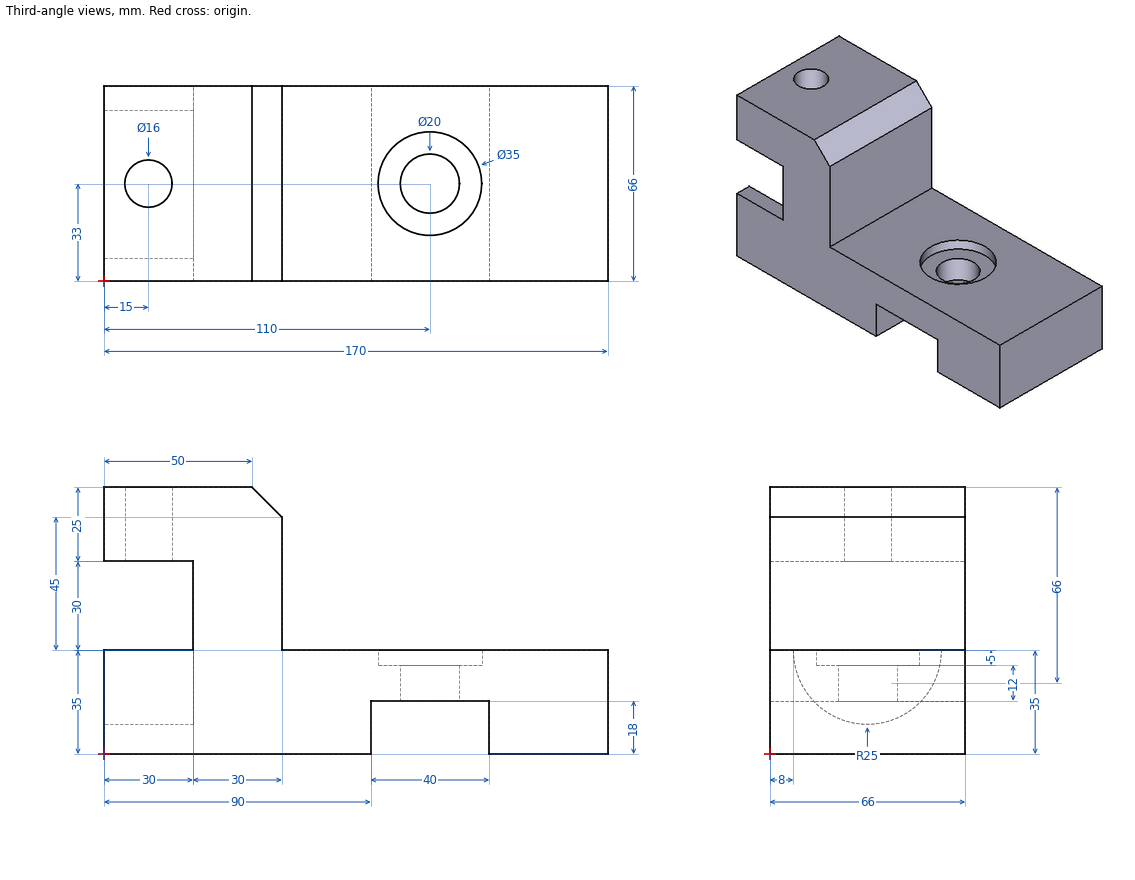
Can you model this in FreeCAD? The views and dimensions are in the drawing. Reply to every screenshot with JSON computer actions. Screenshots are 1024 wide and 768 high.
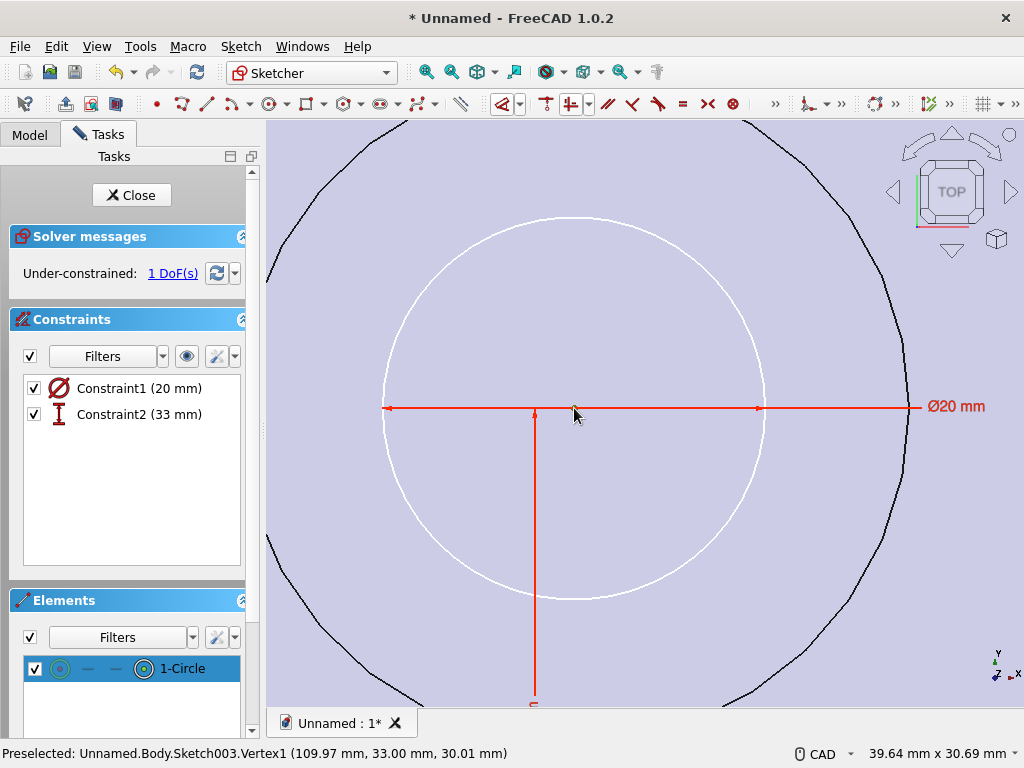
{"action": "key", "text": "l"}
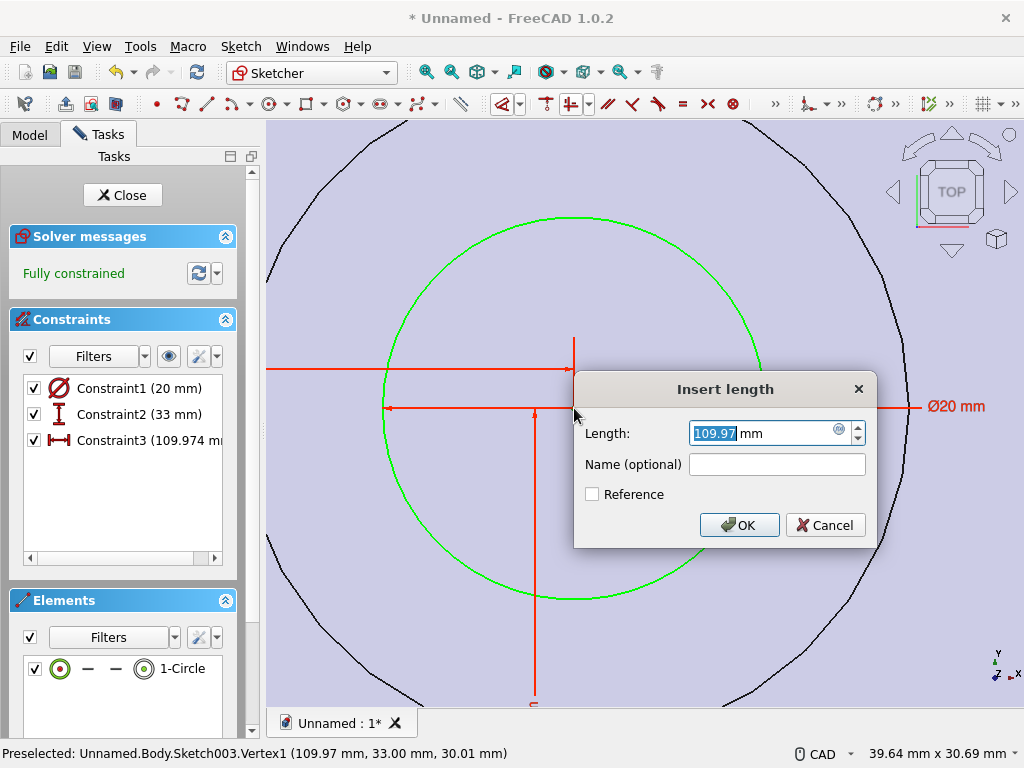
{"action": "type", "text": "110"}
{"action": "key", "text": "Return"}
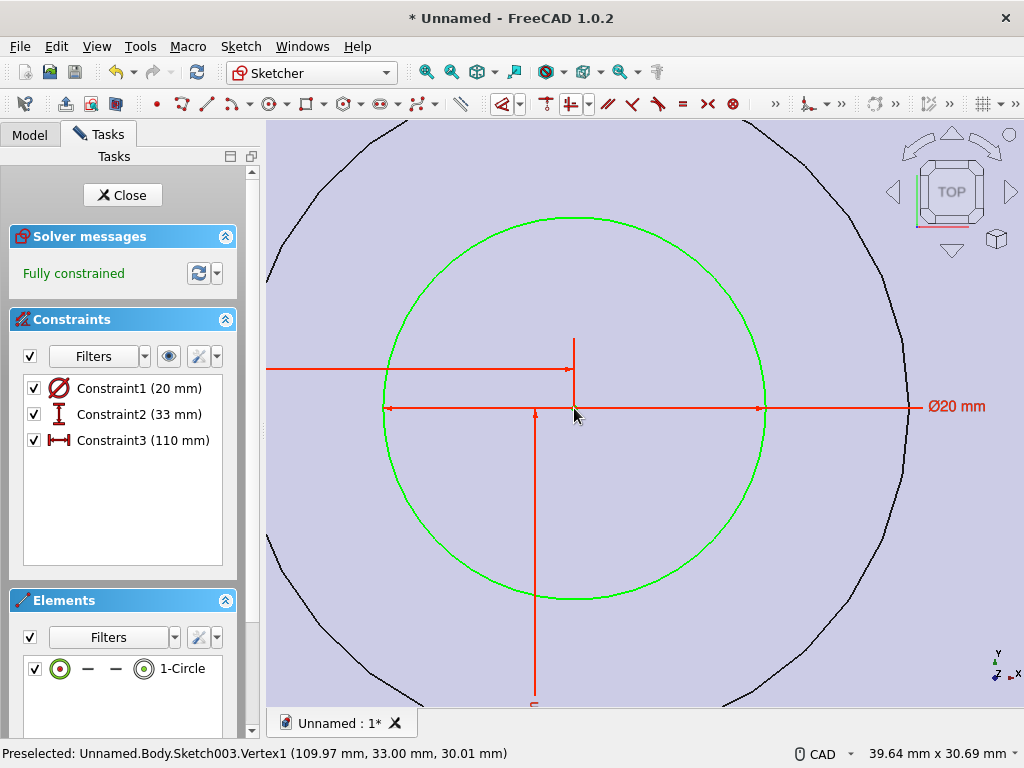
{"action": "left_click", "coordinate": [123, 195]}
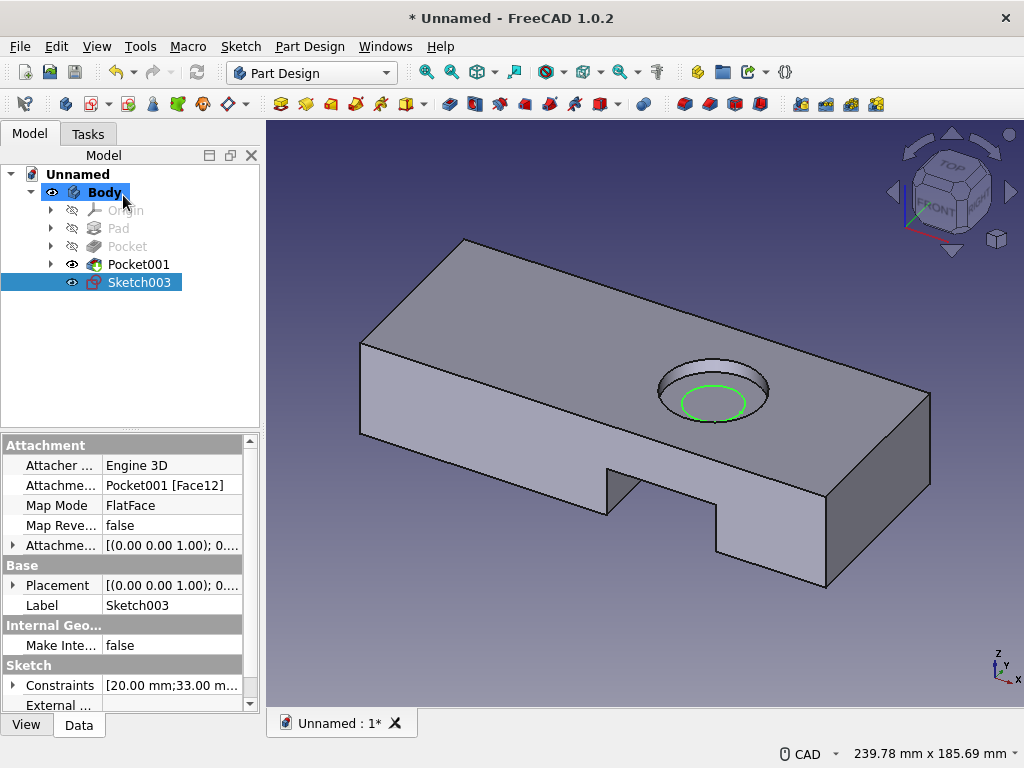
{"action": "left_click", "coordinate": [450, 104]}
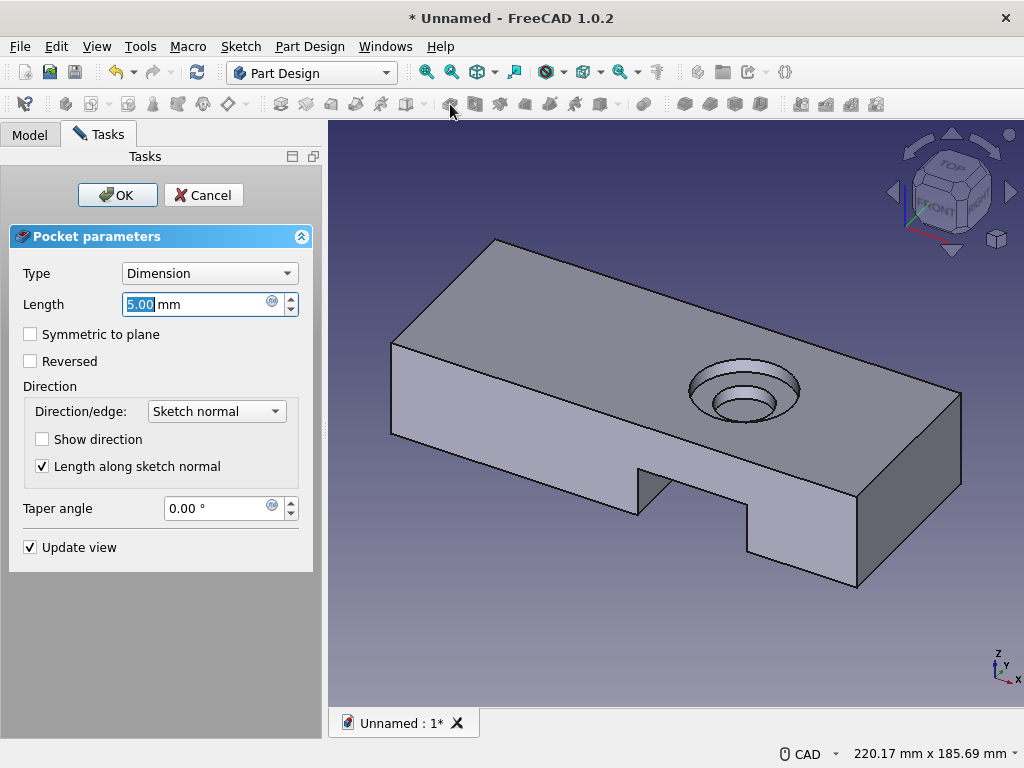
{"action": "type", "text": "12"}
{"action": "key", "text": "Tab"}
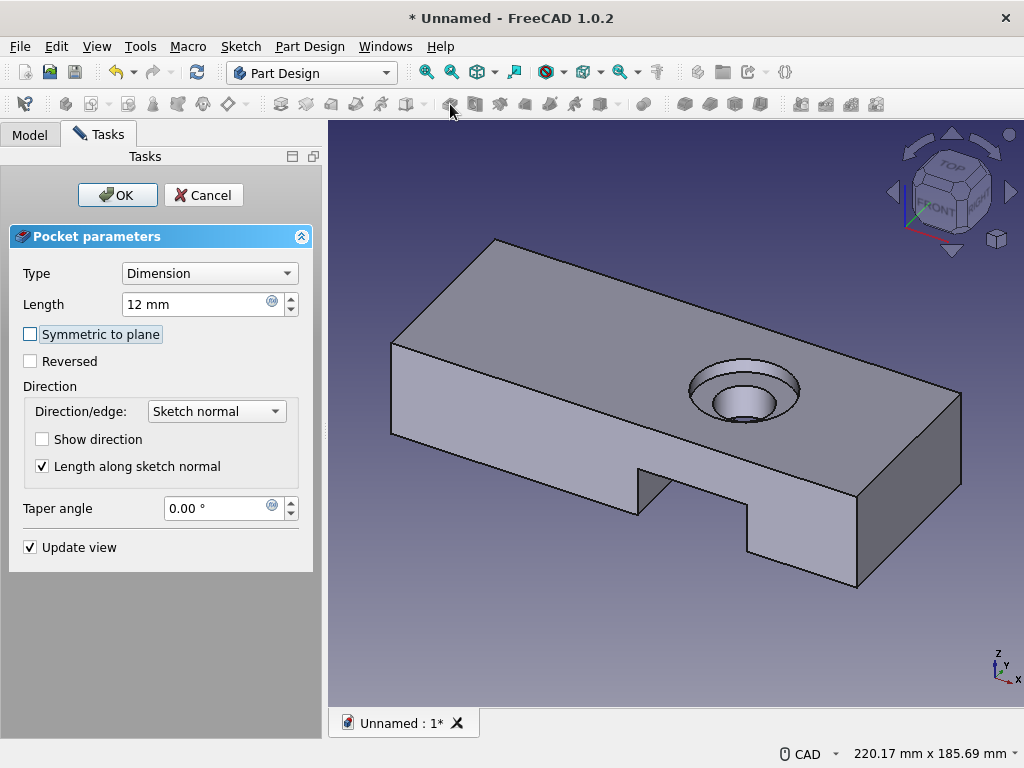
{"action": "left_click", "coordinate": [118, 195]}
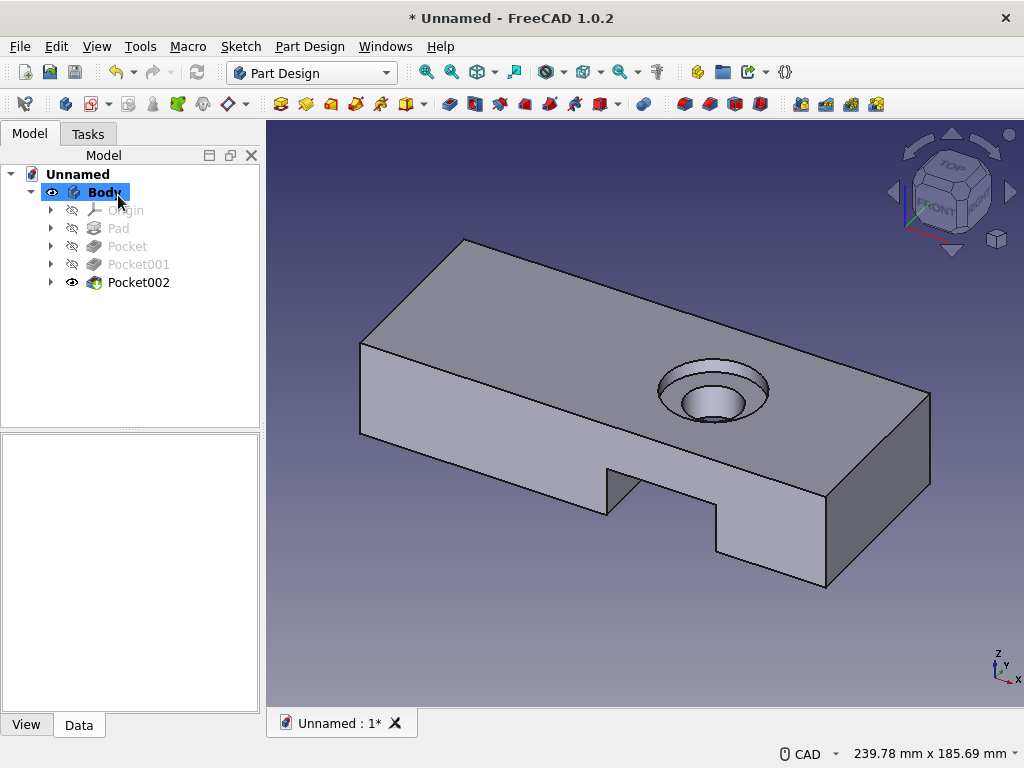
{"action": "left_click", "coordinate": [90, 104]}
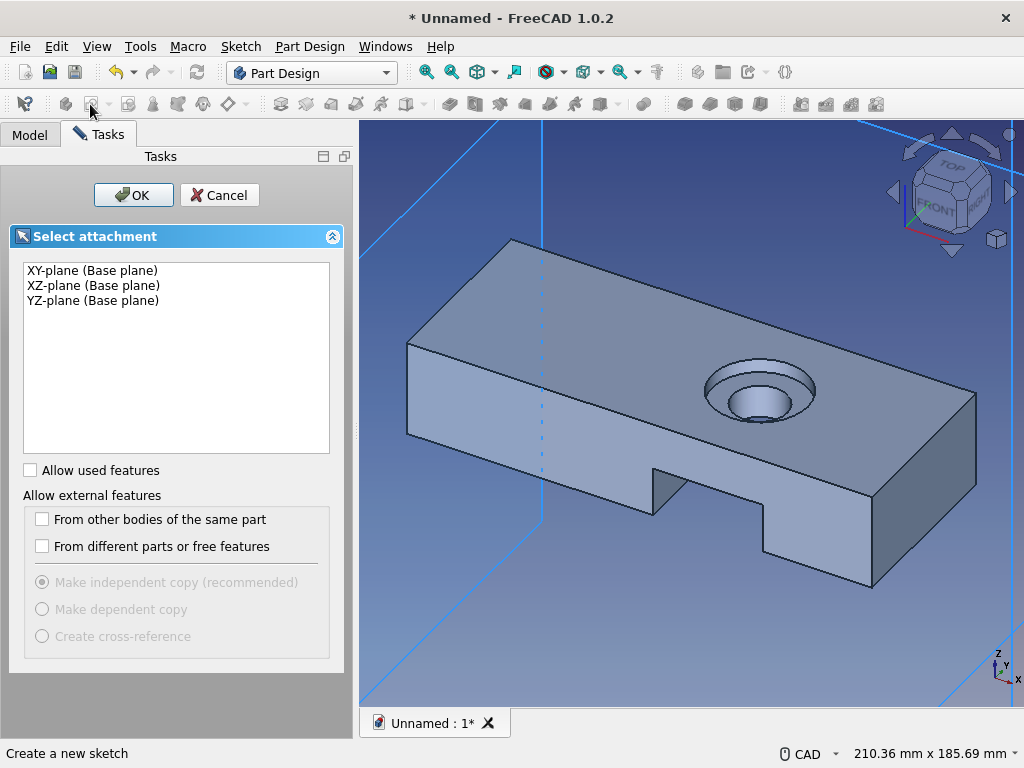
{"action": "left_click", "coordinate": [84, 300]}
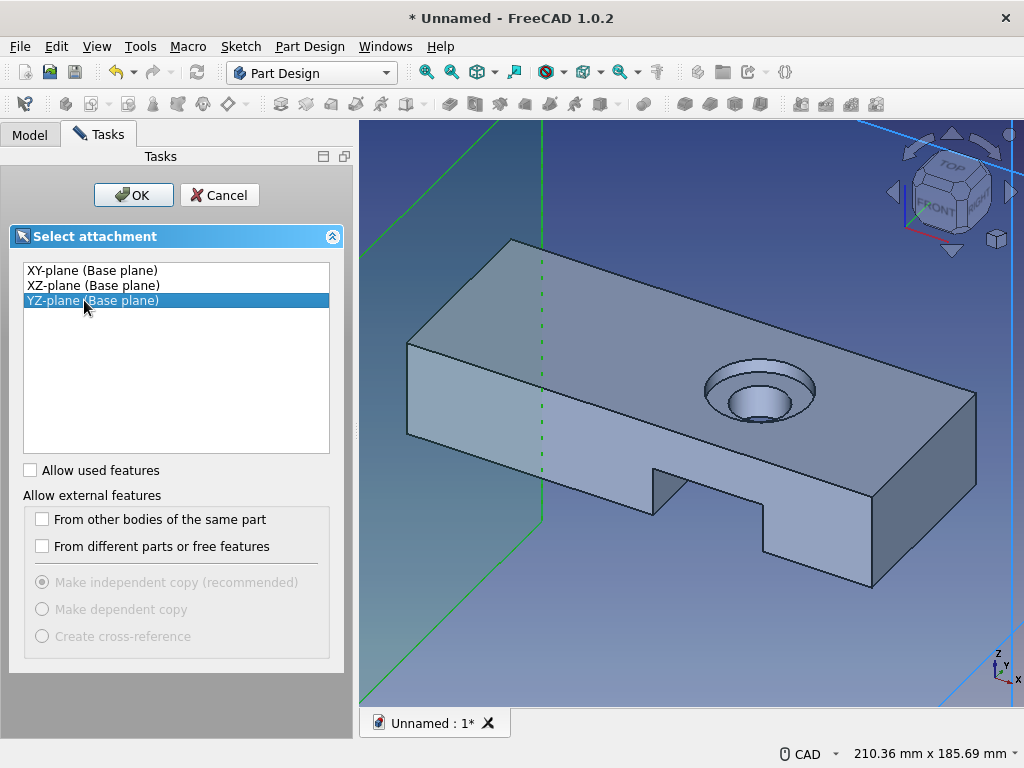
{"action": "left_click", "coordinate": [134, 195]}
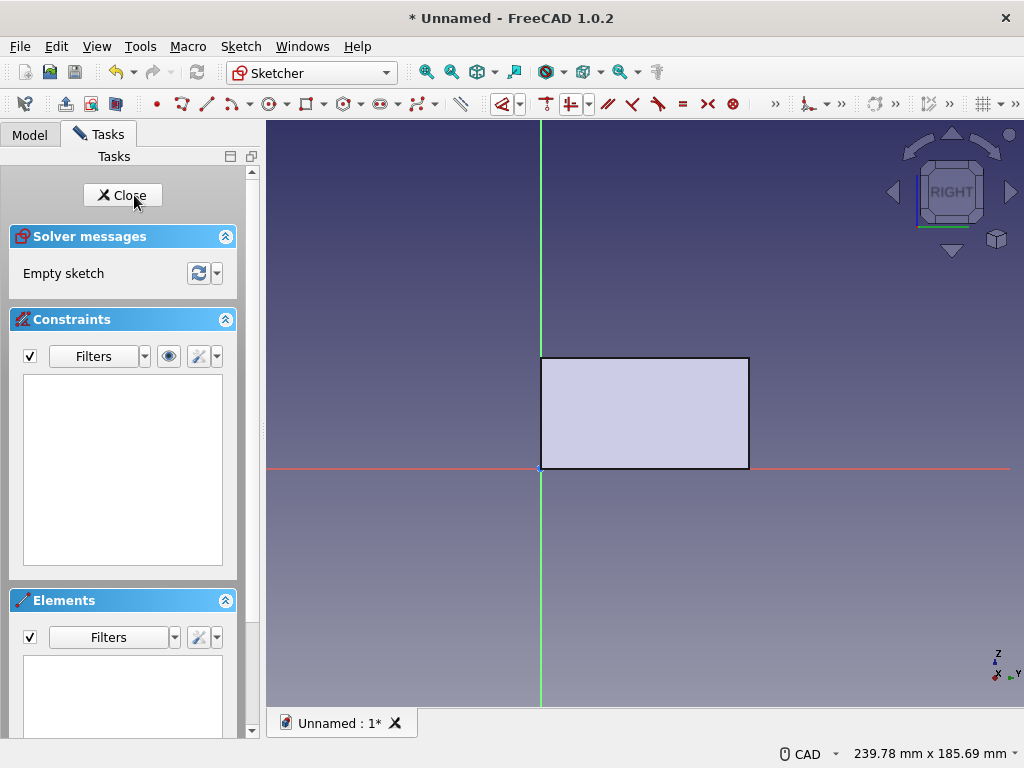
{"action": "key", "text": "q s"}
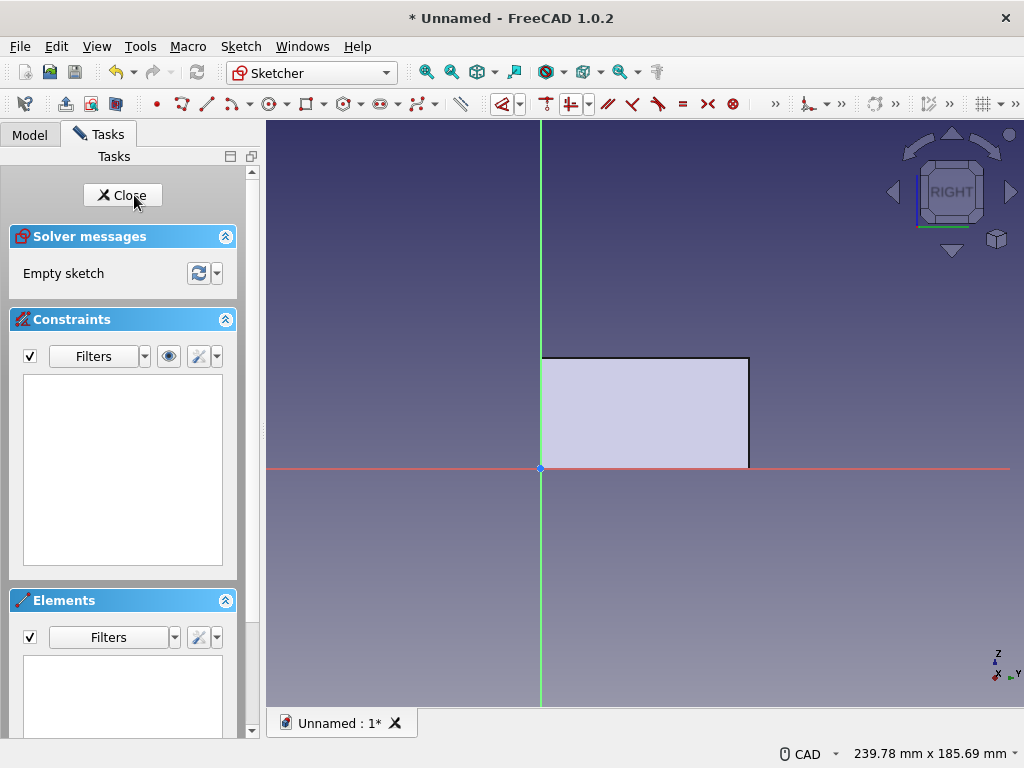
{"action": "scroll", "coordinate": [678, 413], "scroll_direction": "up", "scroll_amount": 4}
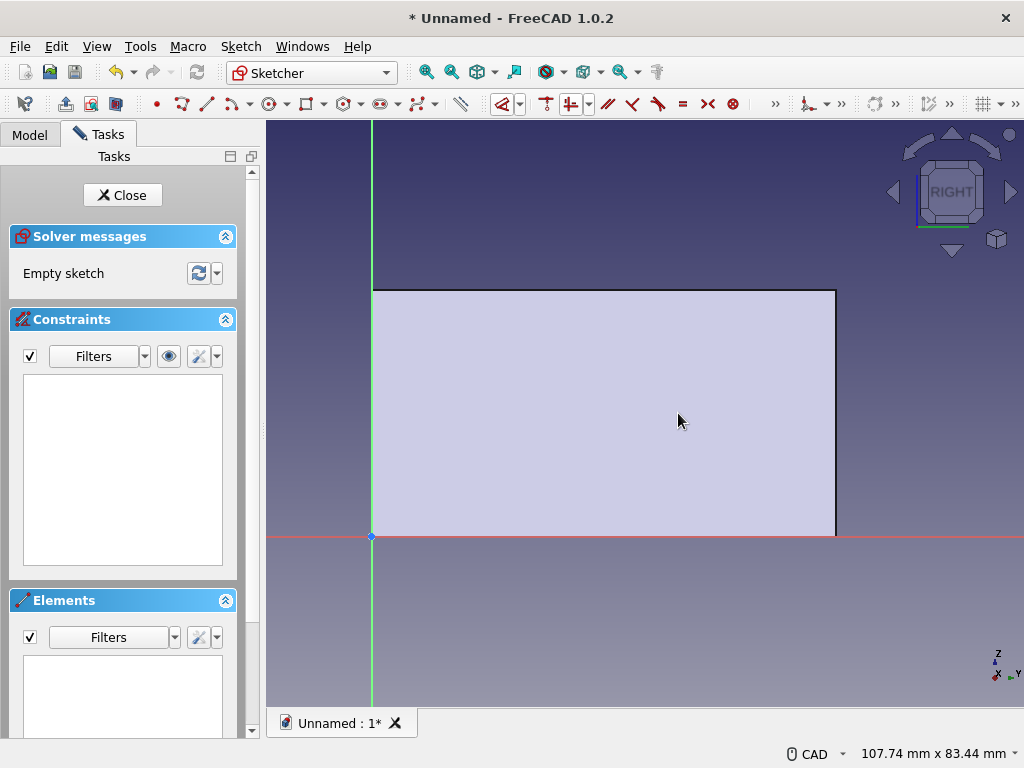
{"action": "key", "text": "g l"}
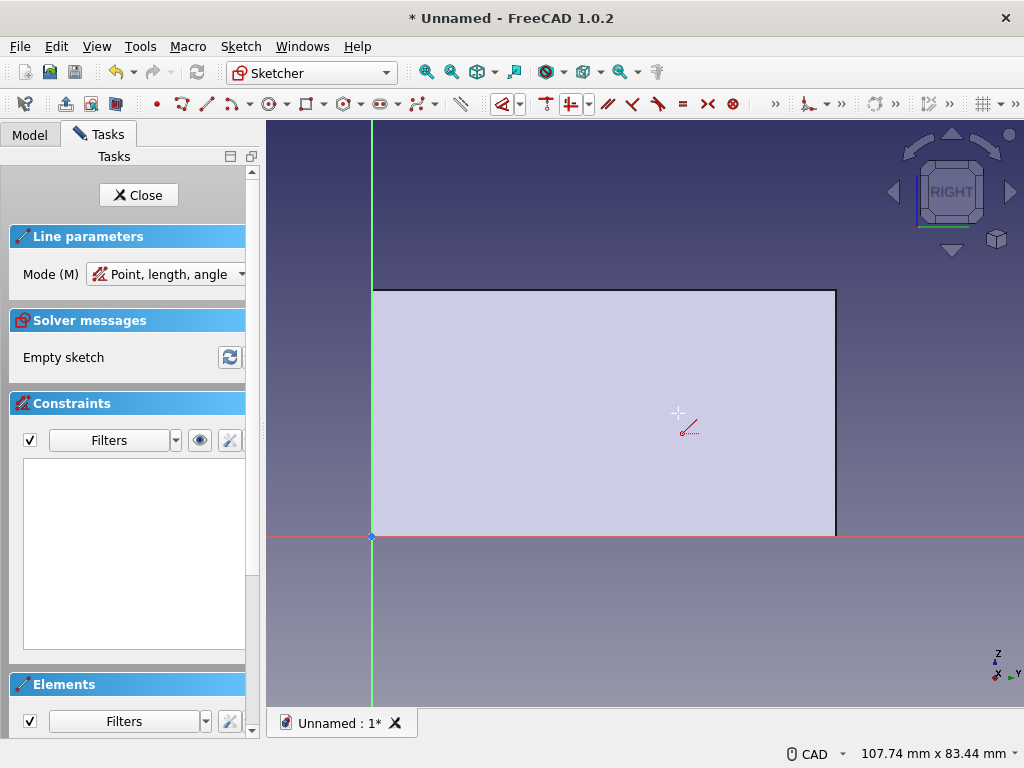
{"action": "left_click", "coordinate": [428, 290]}
{"action": "left_click", "coordinate": [780, 290]}